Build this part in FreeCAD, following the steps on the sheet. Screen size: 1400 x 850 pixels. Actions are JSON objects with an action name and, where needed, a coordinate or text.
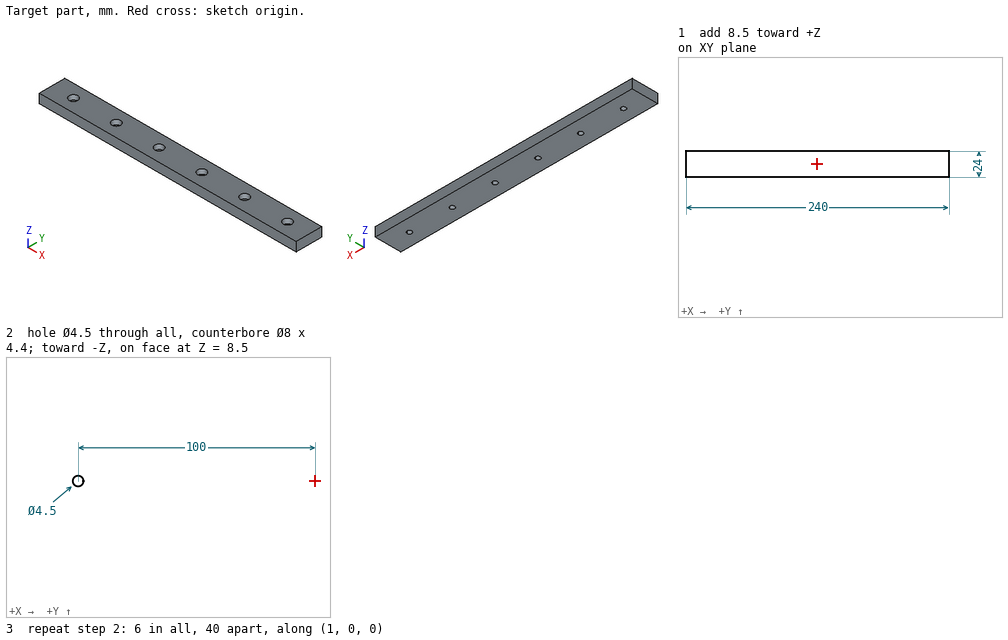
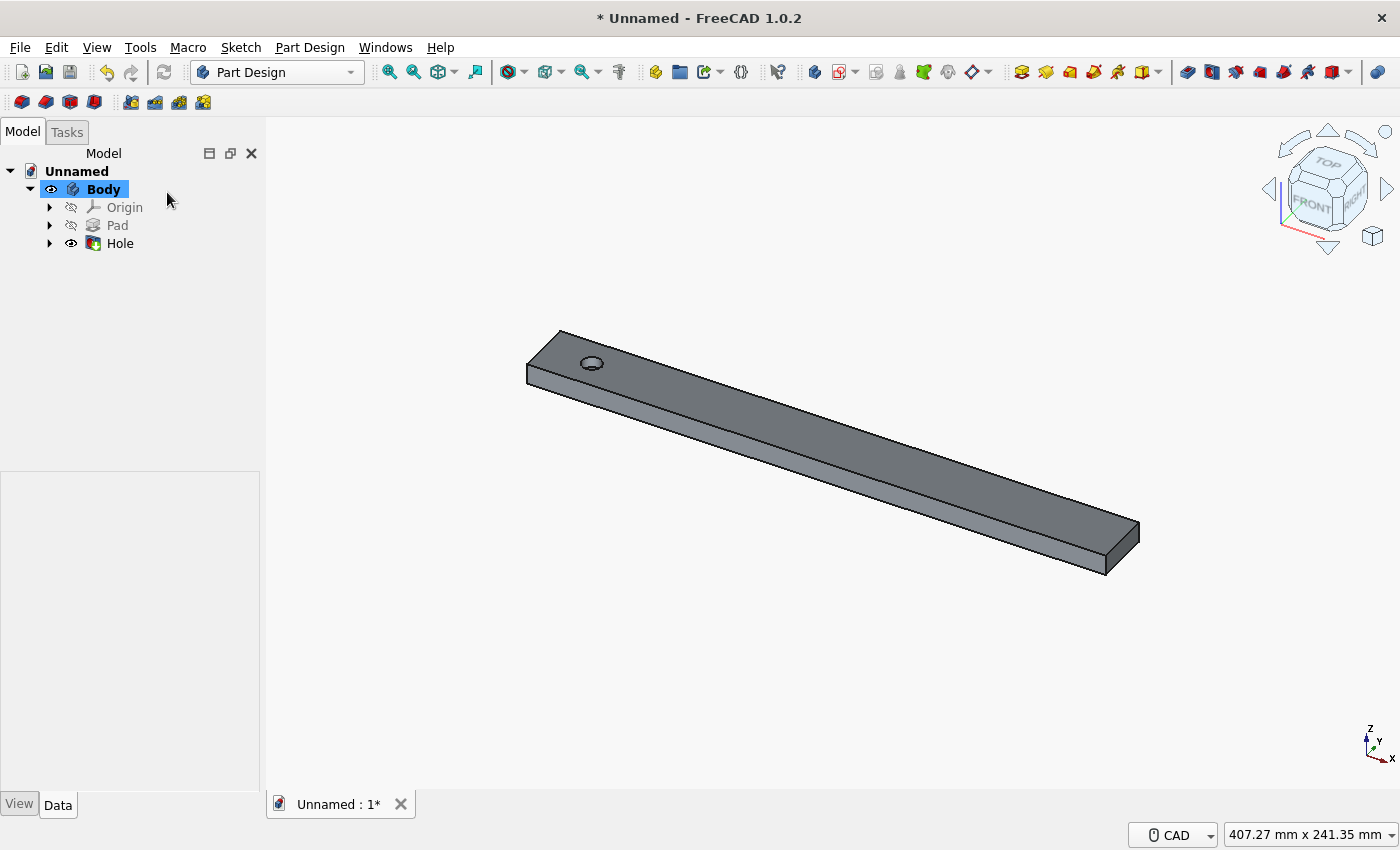
{"action": "left_click", "coordinate": [116, 243]}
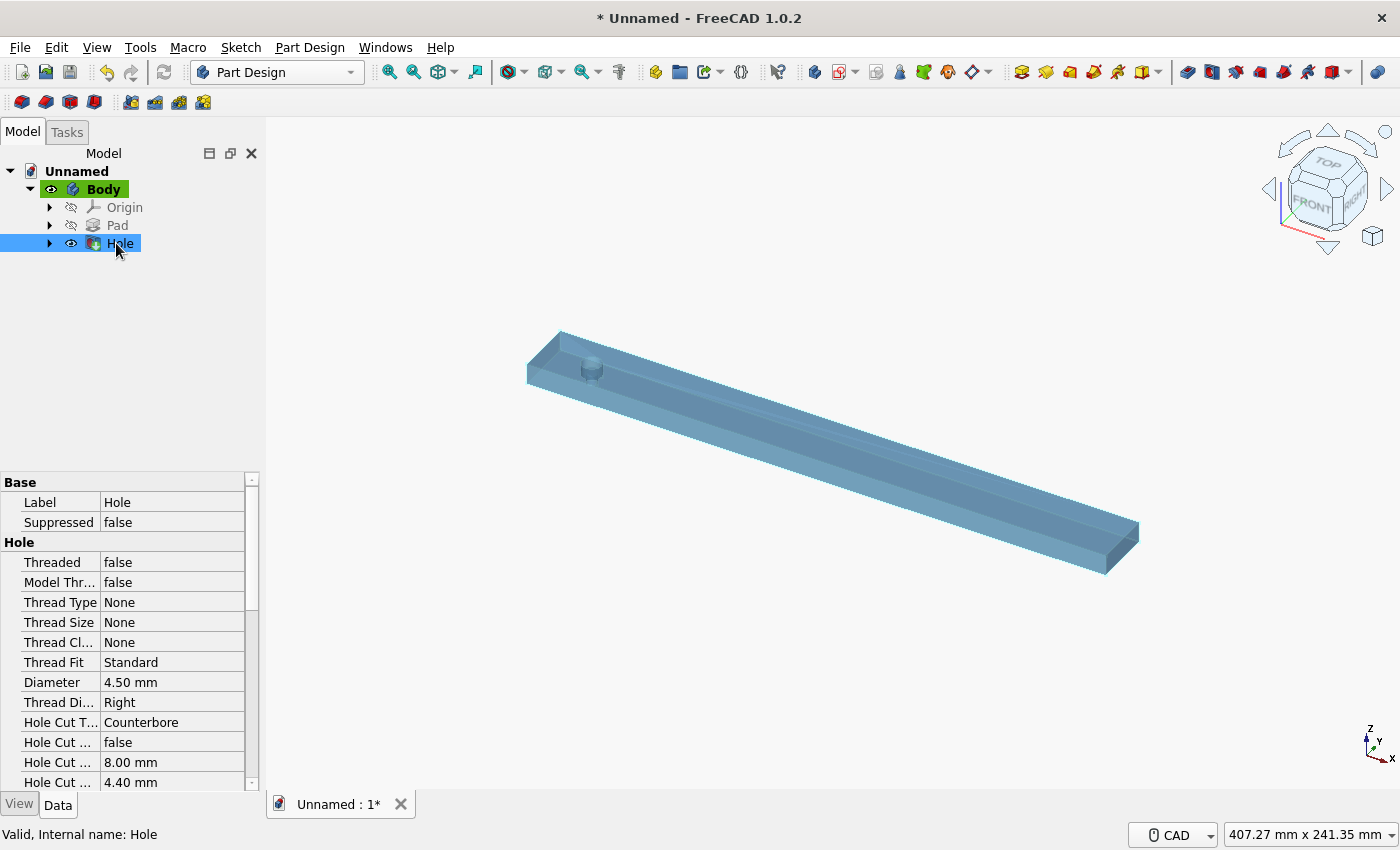
{"action": "left_click", "coordinate": [156, 102]}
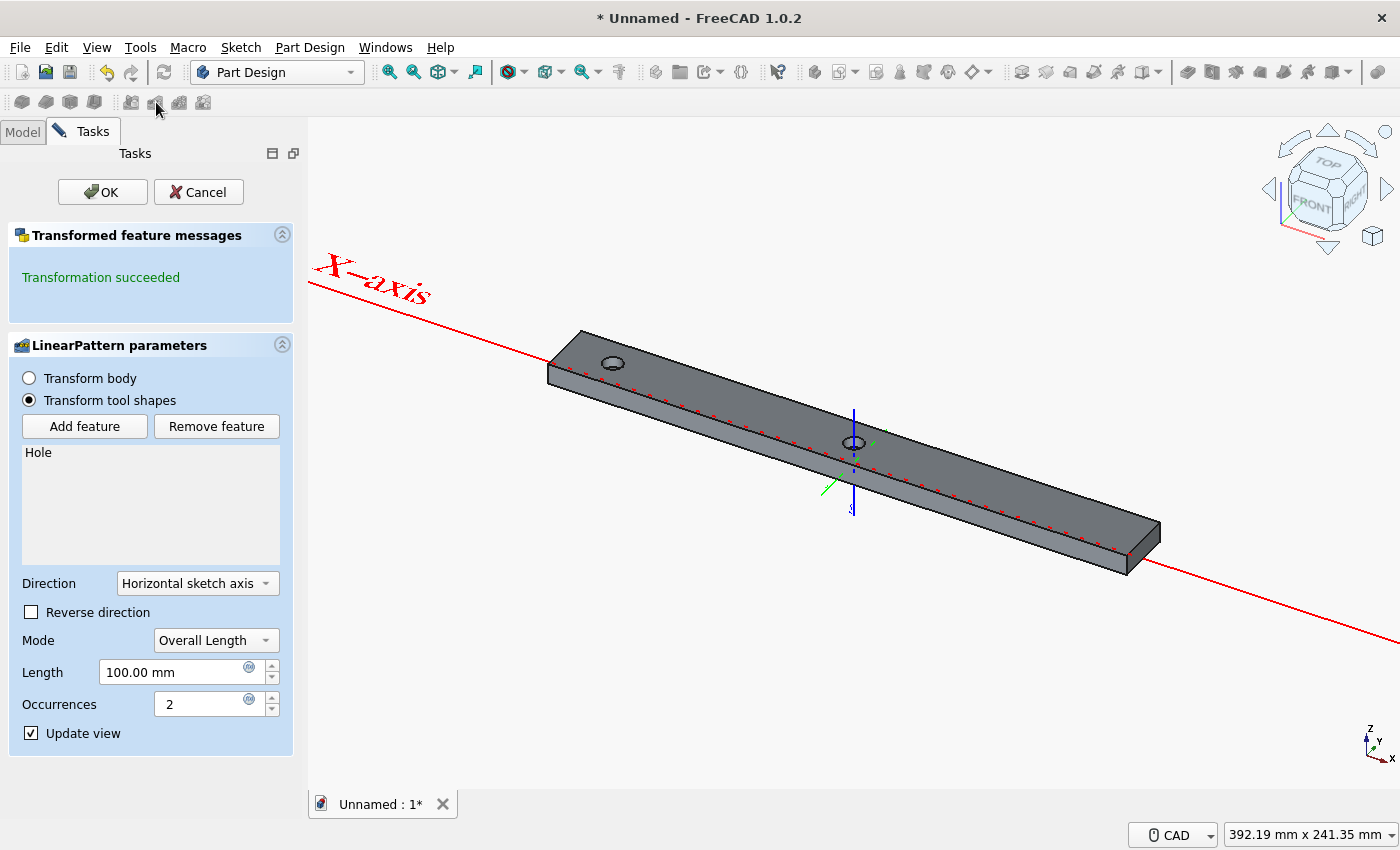
{"action": "left_click", "coordinate": [198, 584]}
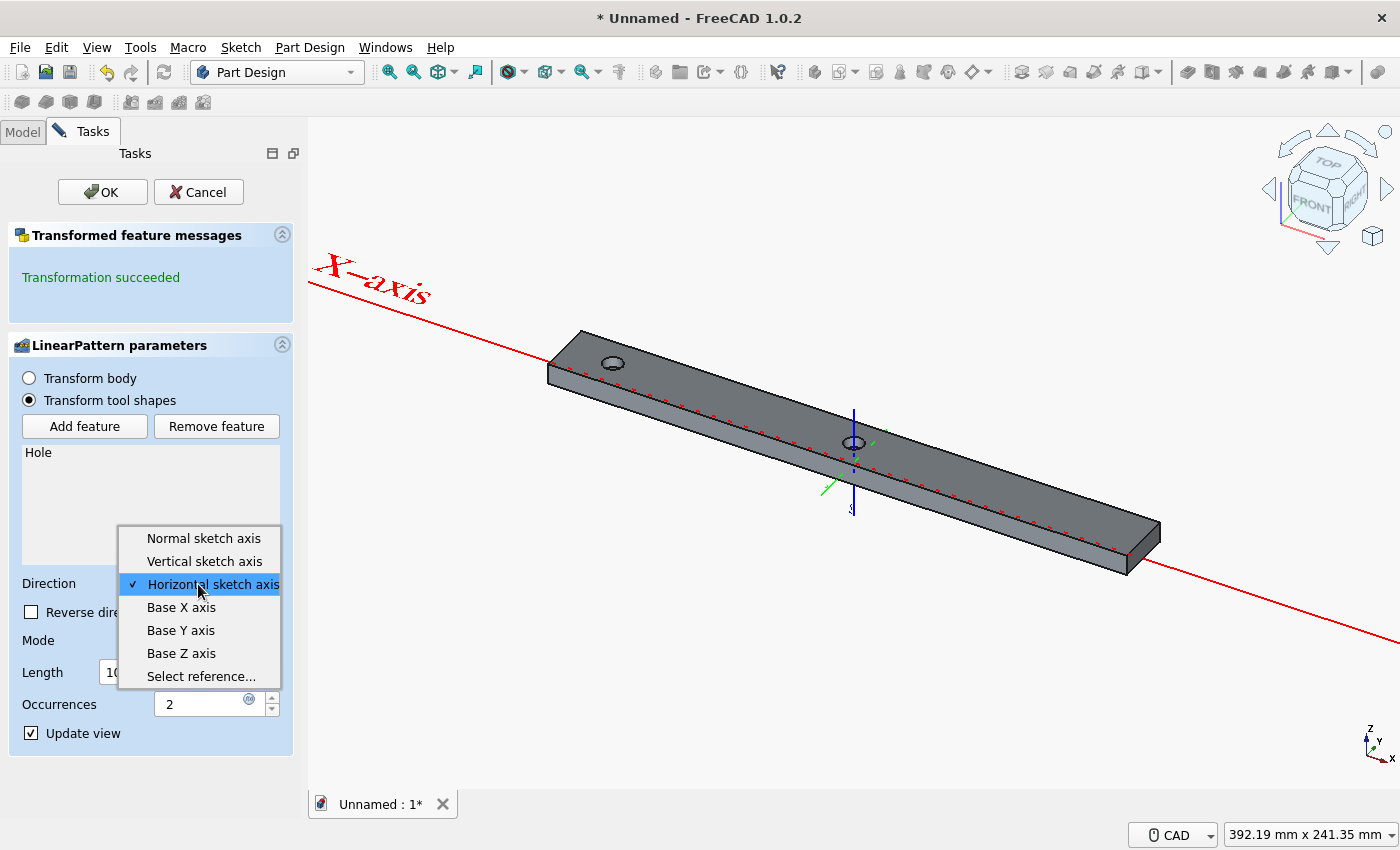
{"action": "left_click", "coordinate": [198, 608]}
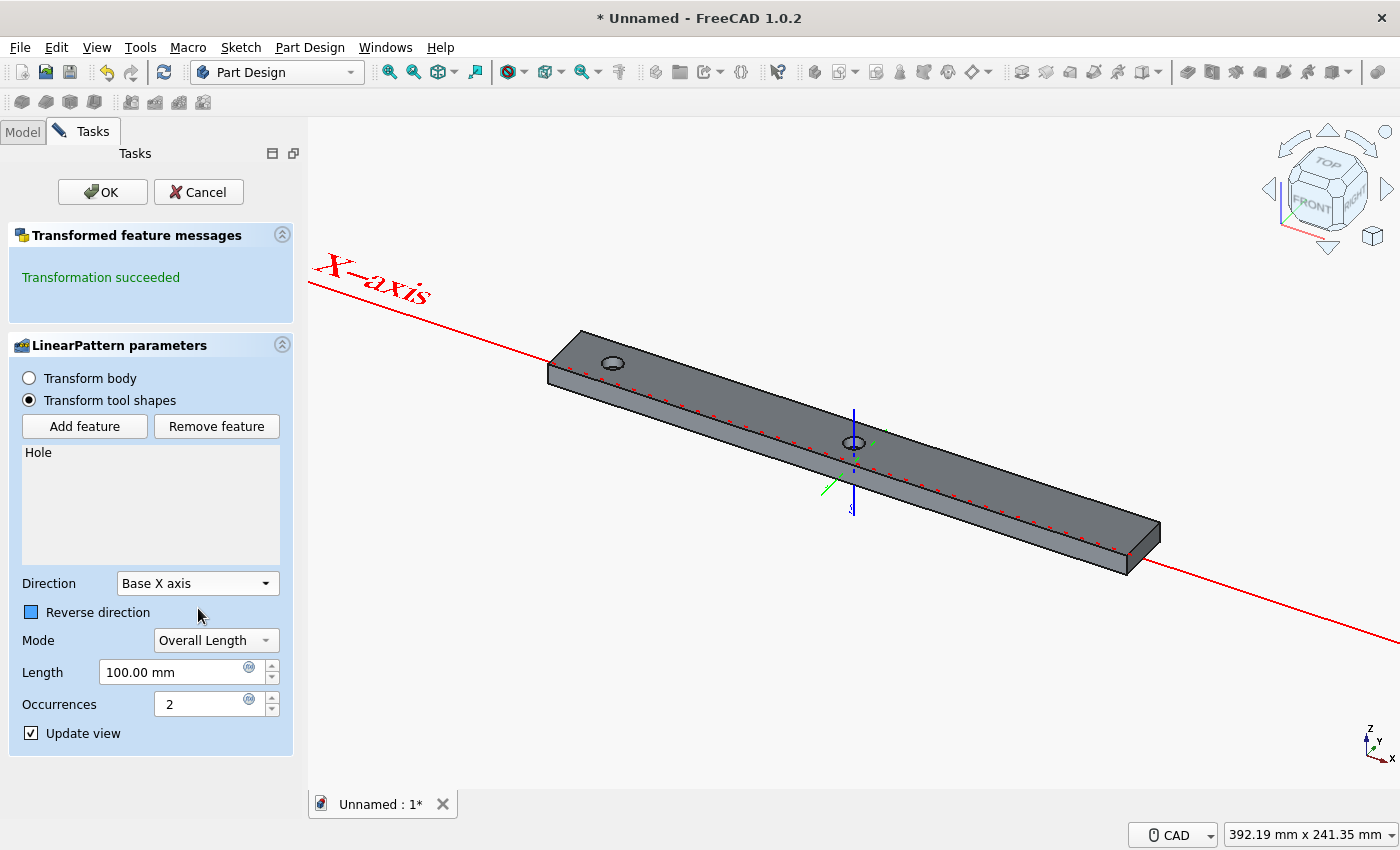
{"action": "left_click", "coordinate": [217, 640]}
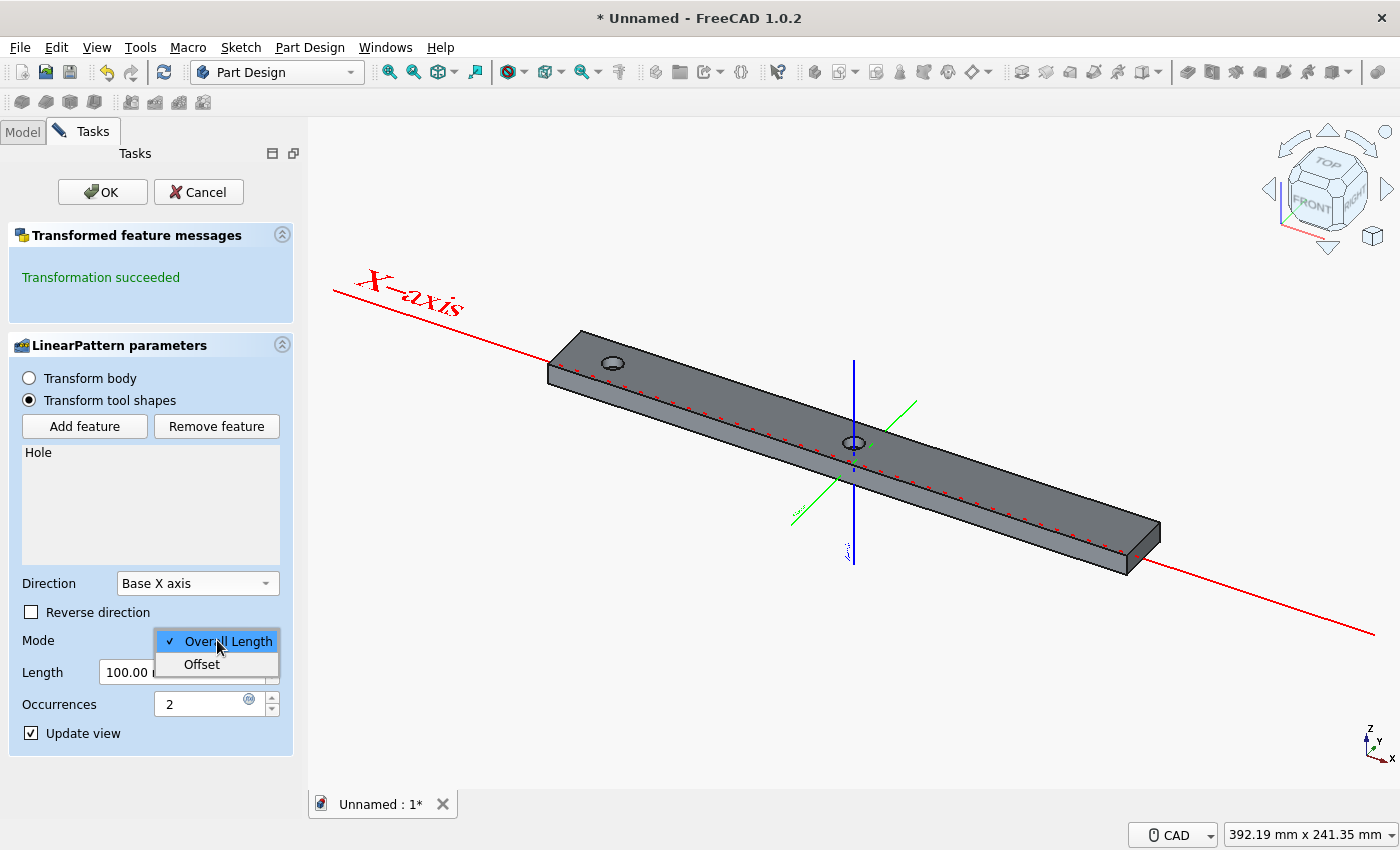
{"action": "left_click", "coordinate": [216, 664]}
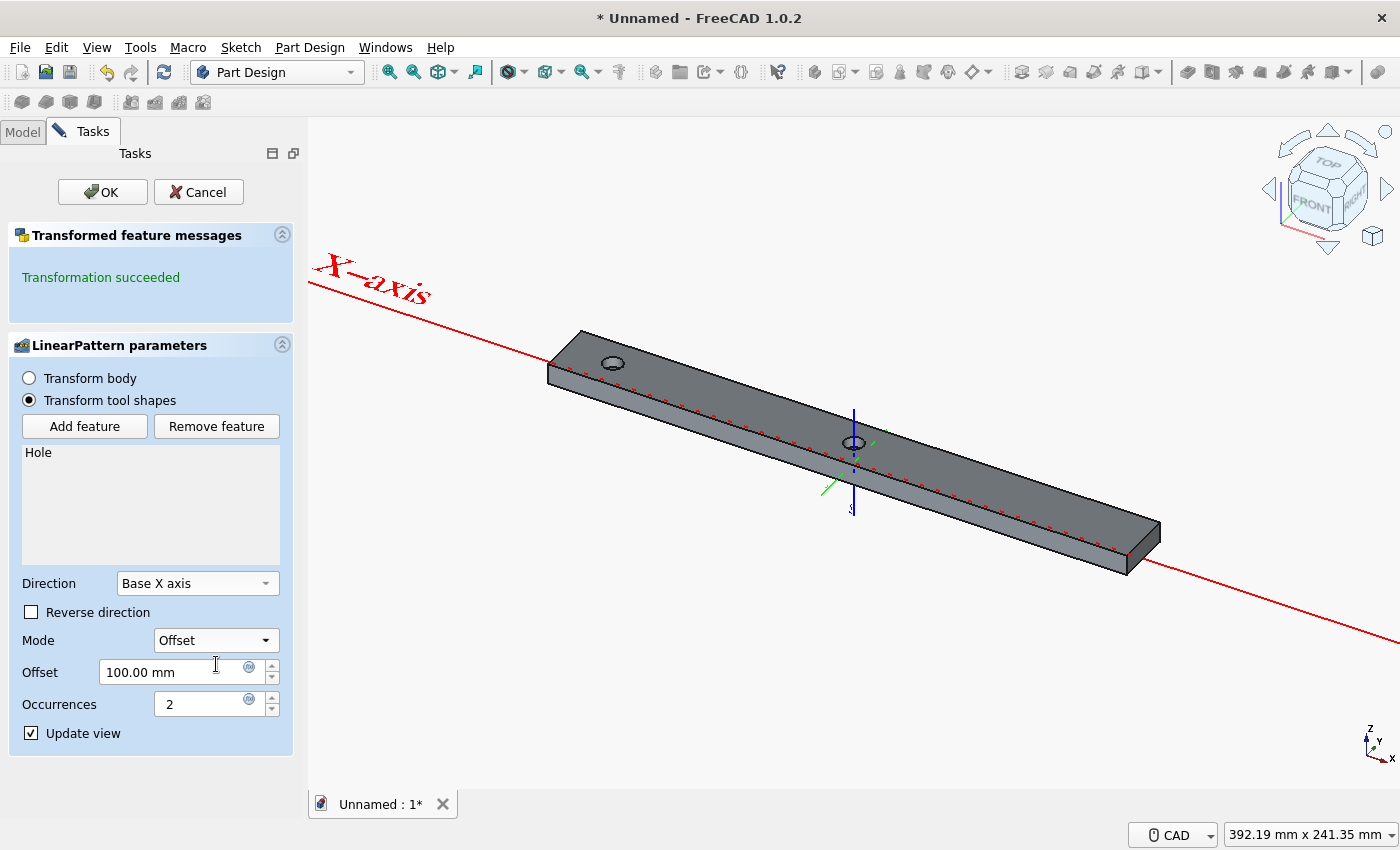
{"action": "triple_click", "coordinate": [182, 672]}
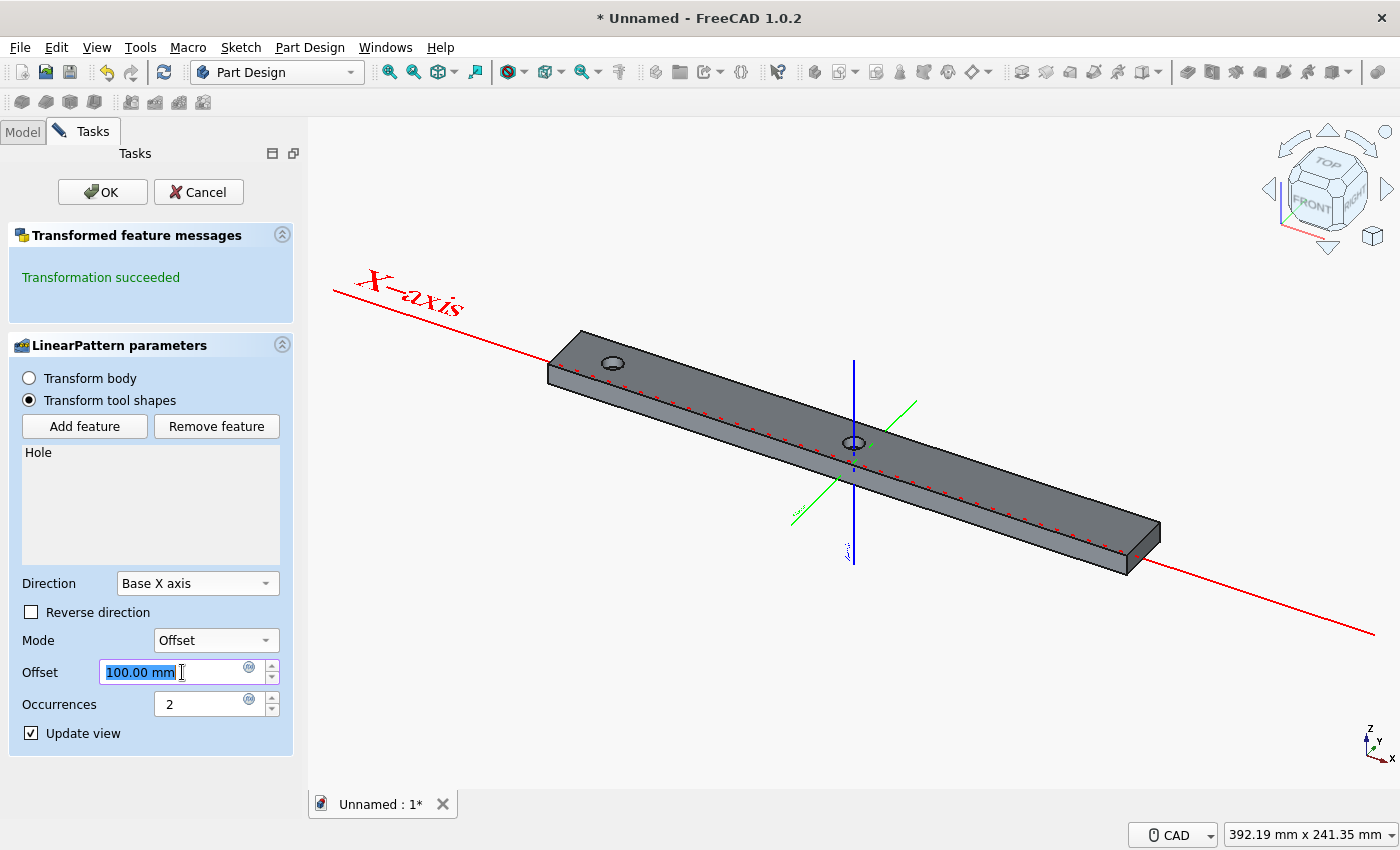
{"action": "type", "text": "40"}
{"action": "key", "text": "Tab"}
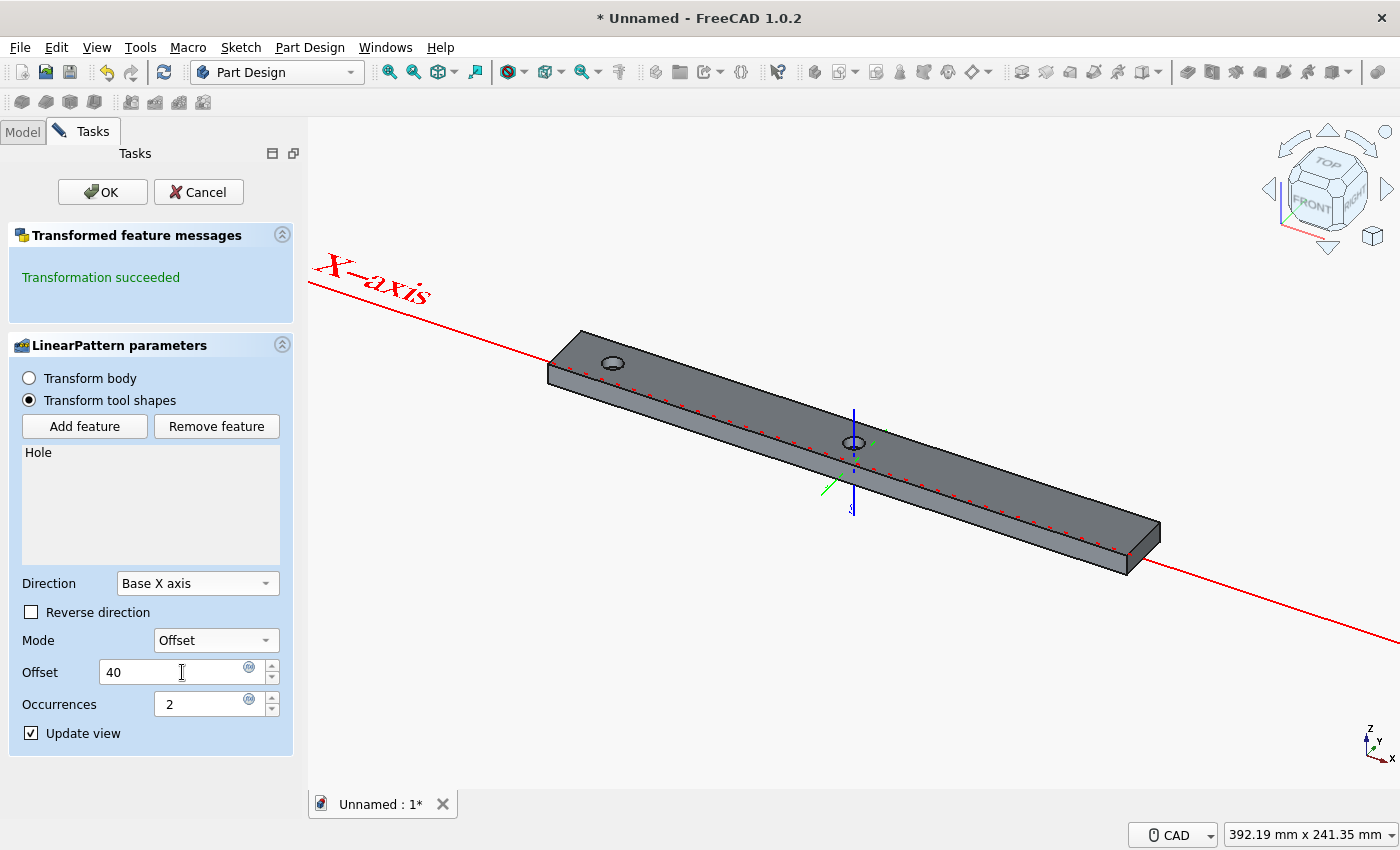
{"action": "triple_click", "coordinate": [209, 704]}